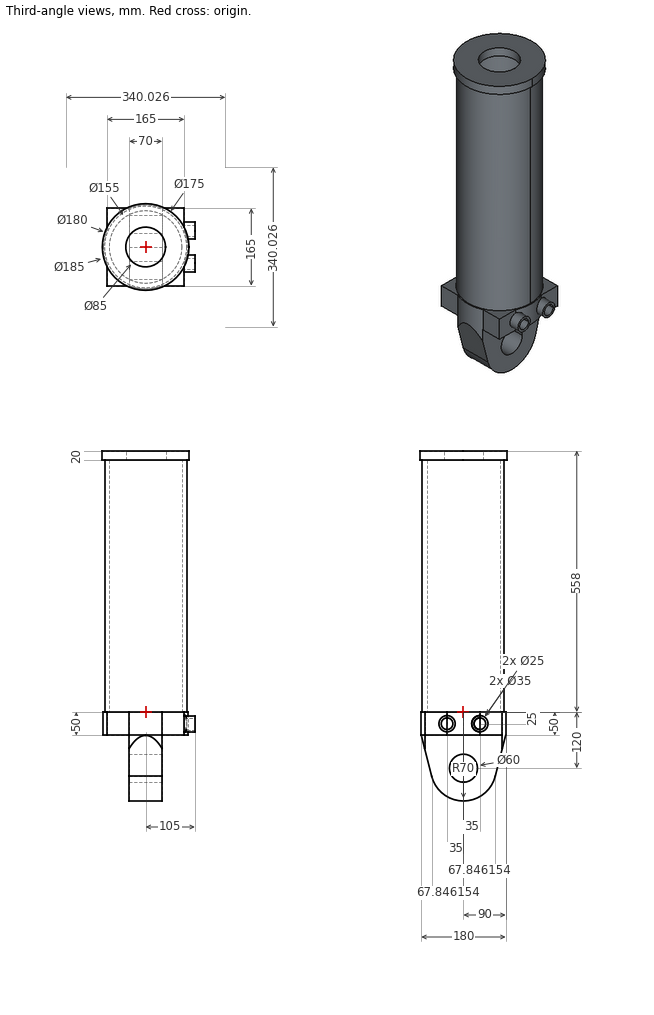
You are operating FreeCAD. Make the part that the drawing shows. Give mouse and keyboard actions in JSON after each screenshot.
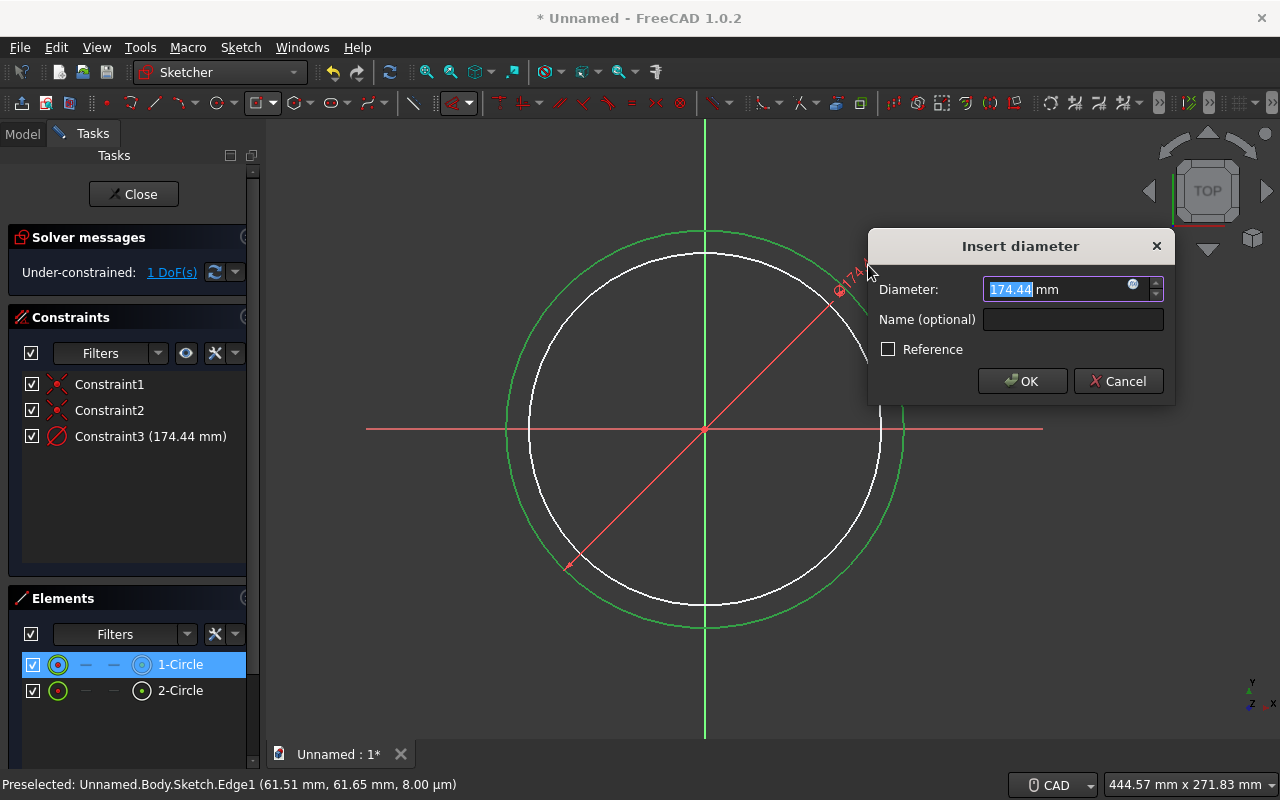
{"action": "type", "text": "175"}
{"action": "key", "text": "Return"}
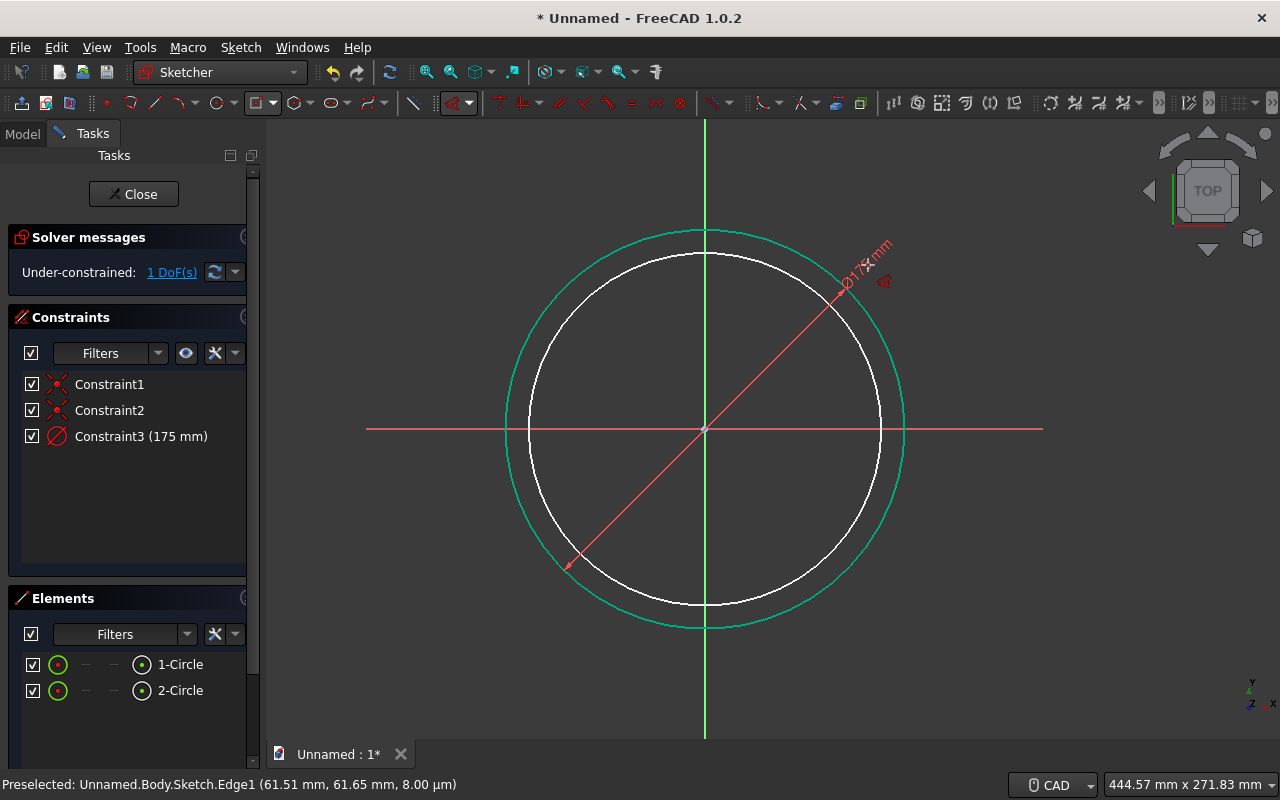
{"action": "left_click", "coordinate": [829, 304]}
{"action": "left_click", "coordinate": [927, 363]}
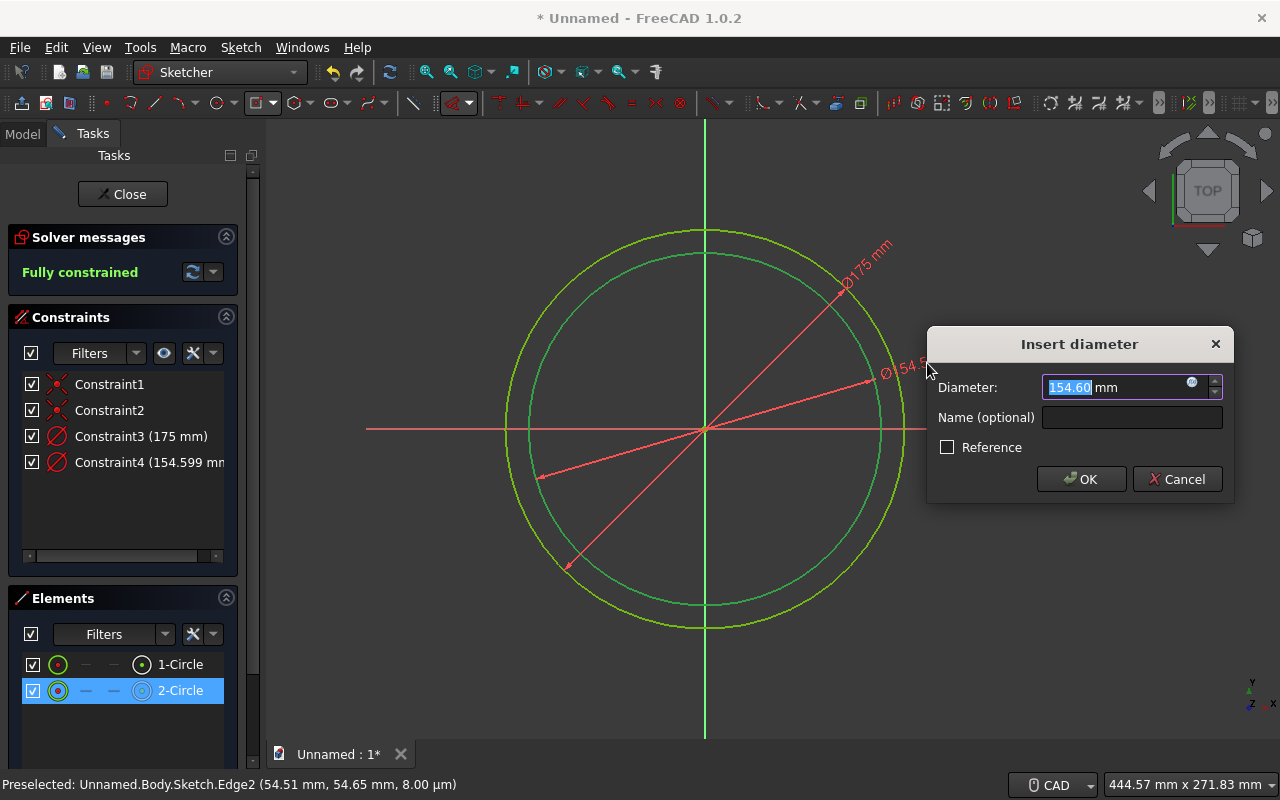
{"action": "type", "text": "155"}
{"action": "key", "text": "Return"}
{"action": "key", "text": "Escape"}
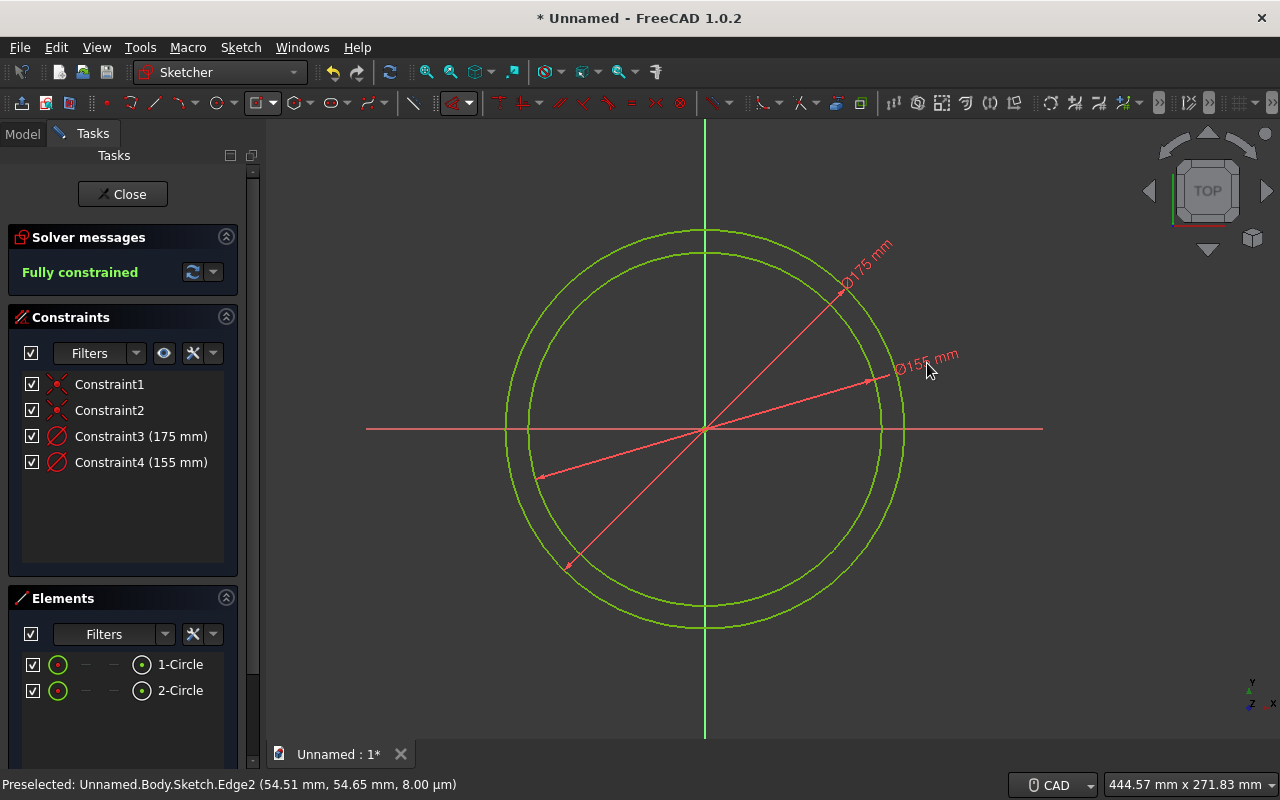
{"action": "left_click", "coordinate": [123, 194]}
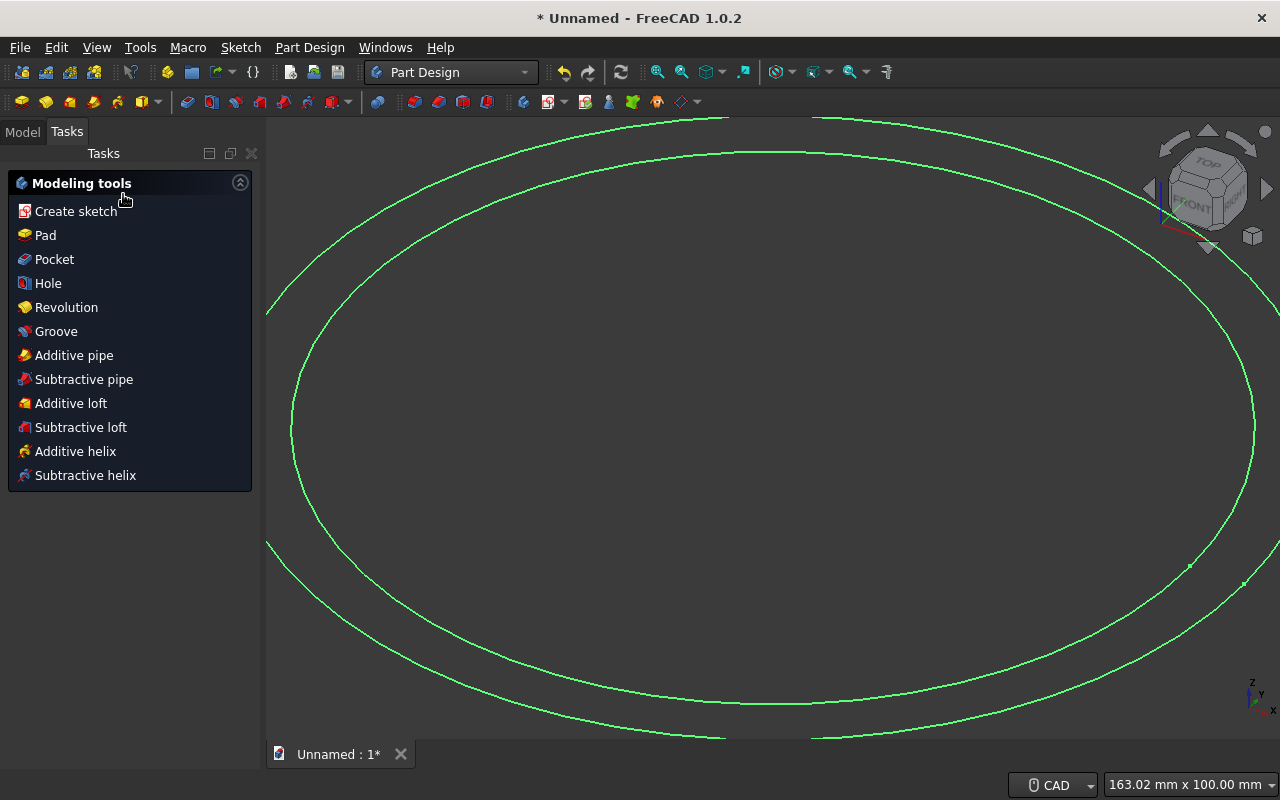
{"action": "left_click", "coordinate": [22, 102]}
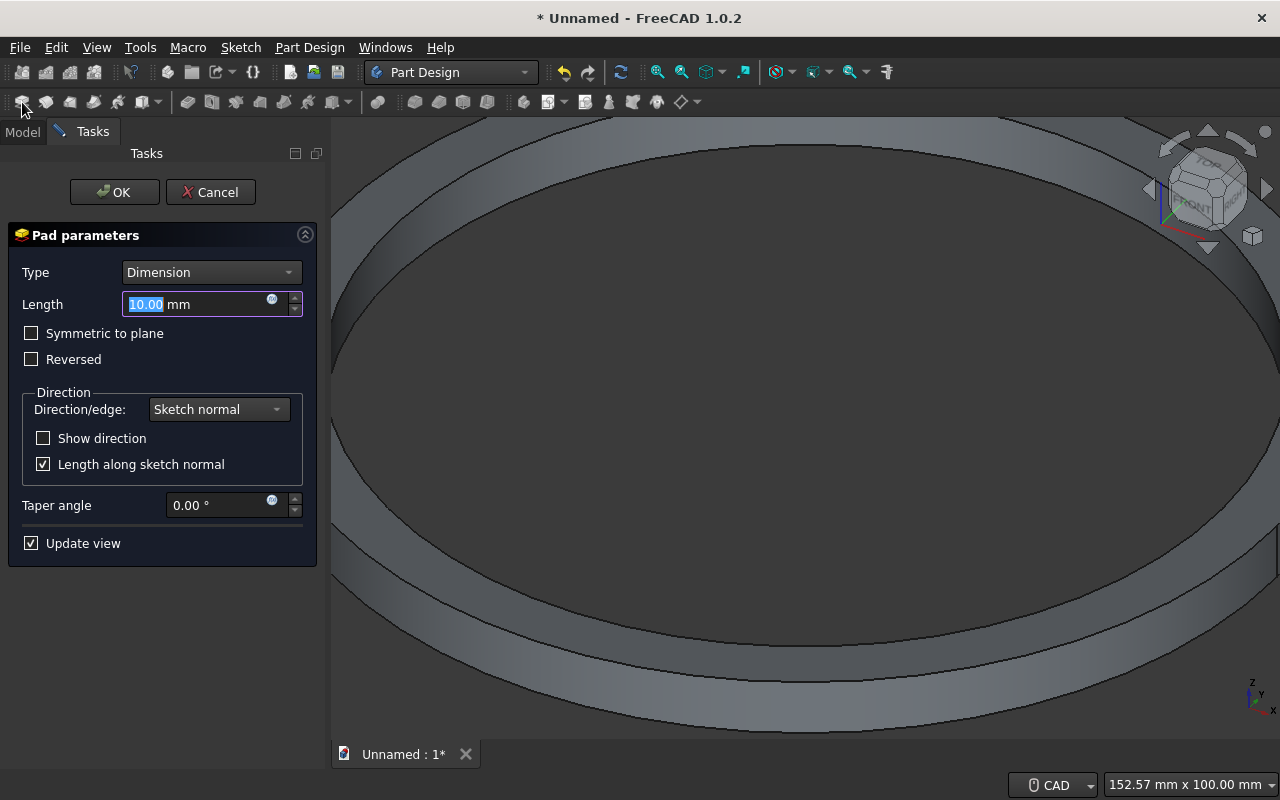
{"action": "type", "text": "558"}
{"action": "key", "text": "Tab"}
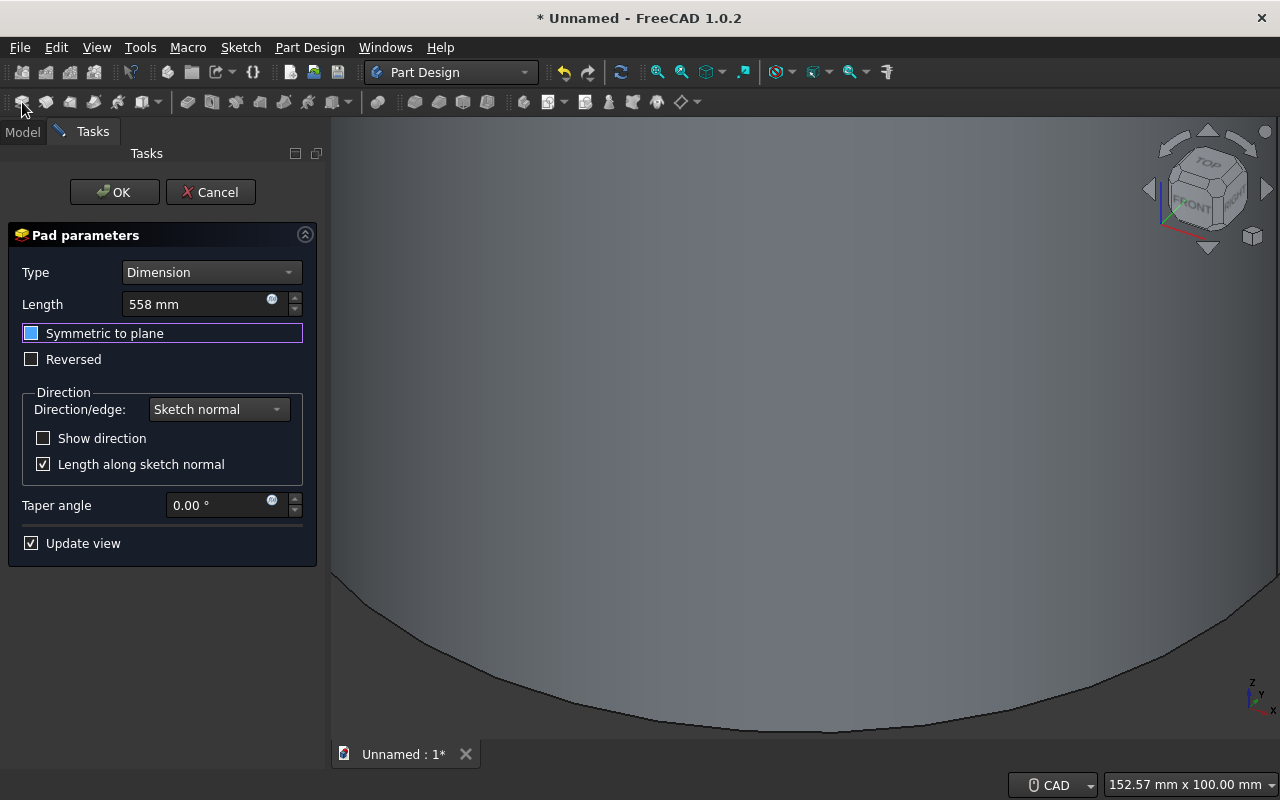
{"action": "left_click", "coordinate": [115, 192]}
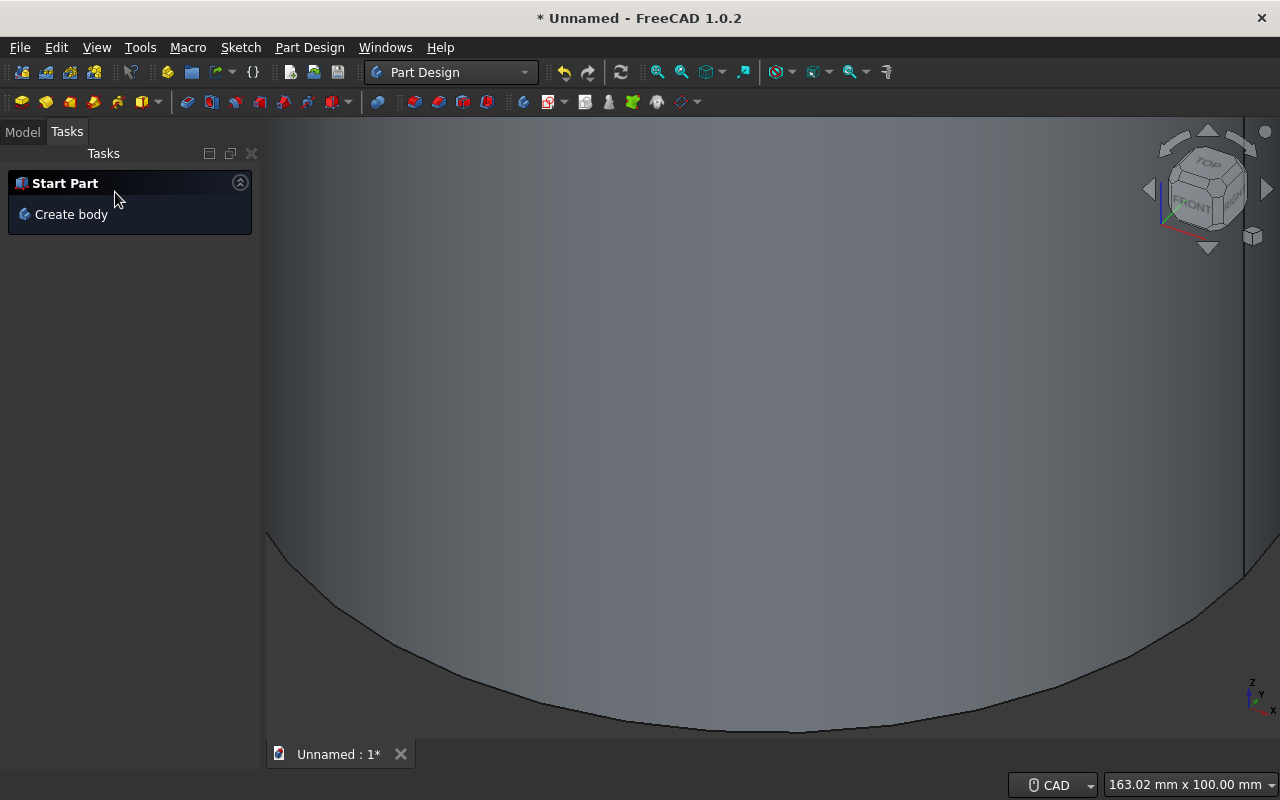
{"action": "key", "text": "v f"}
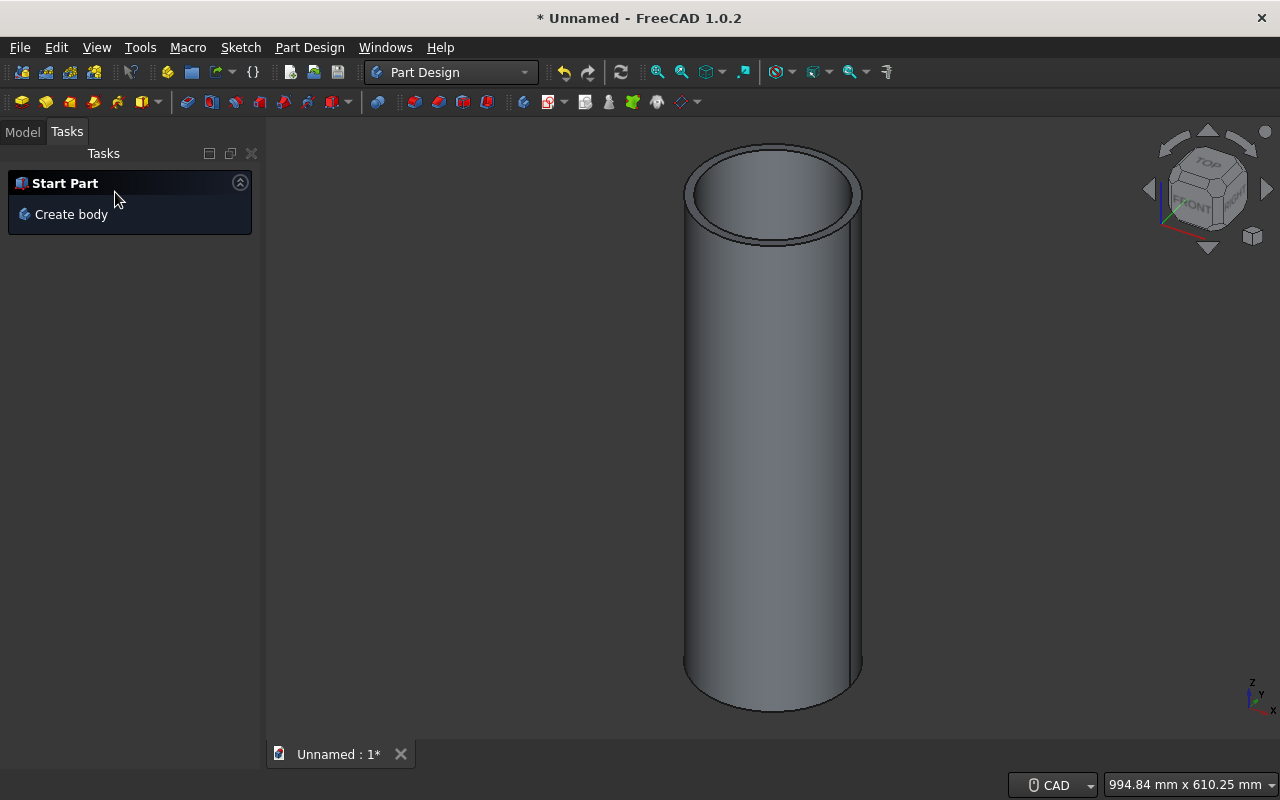
{"action": "left_click", "coordinate": [548, 102]}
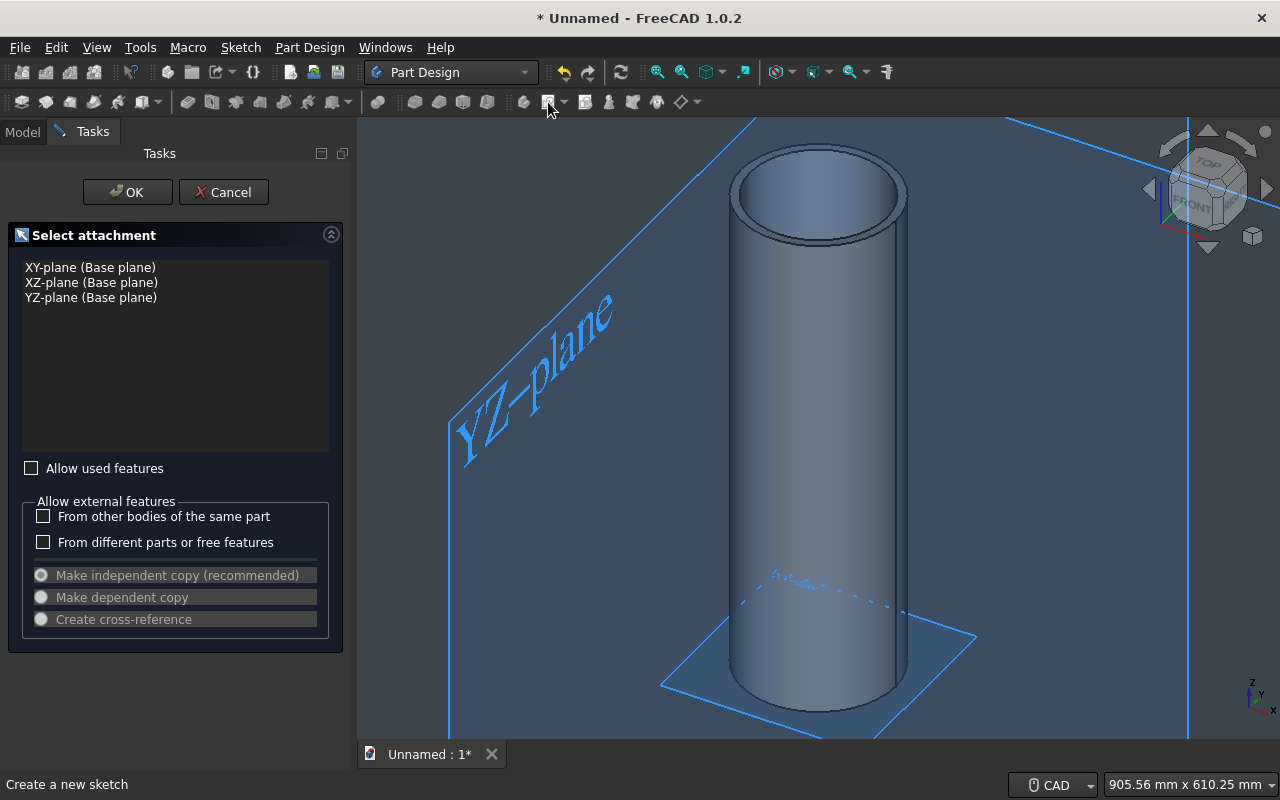
{"action": "left_click", "coordinate": [82, 268]}